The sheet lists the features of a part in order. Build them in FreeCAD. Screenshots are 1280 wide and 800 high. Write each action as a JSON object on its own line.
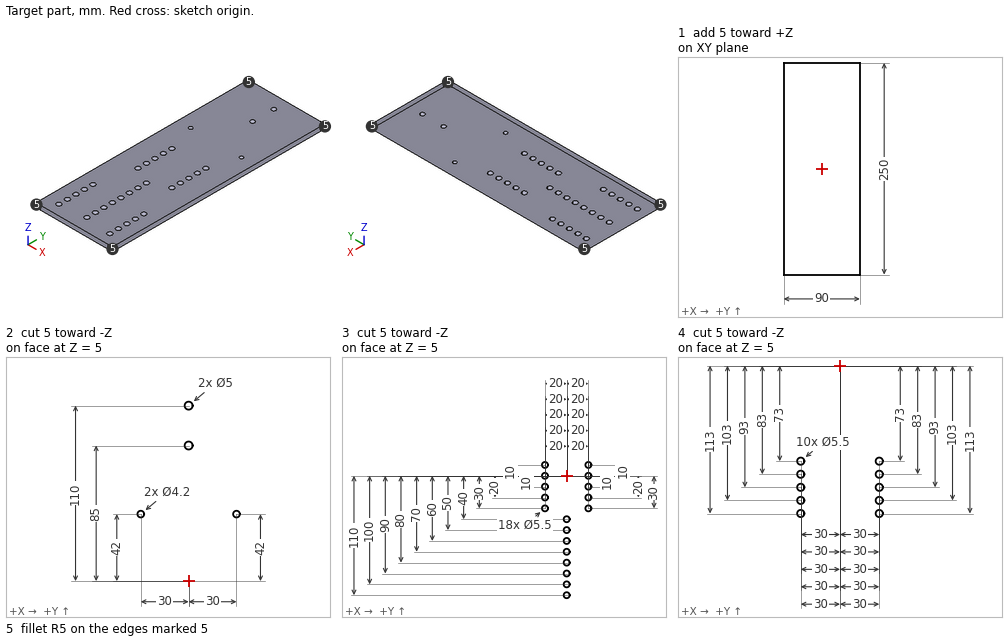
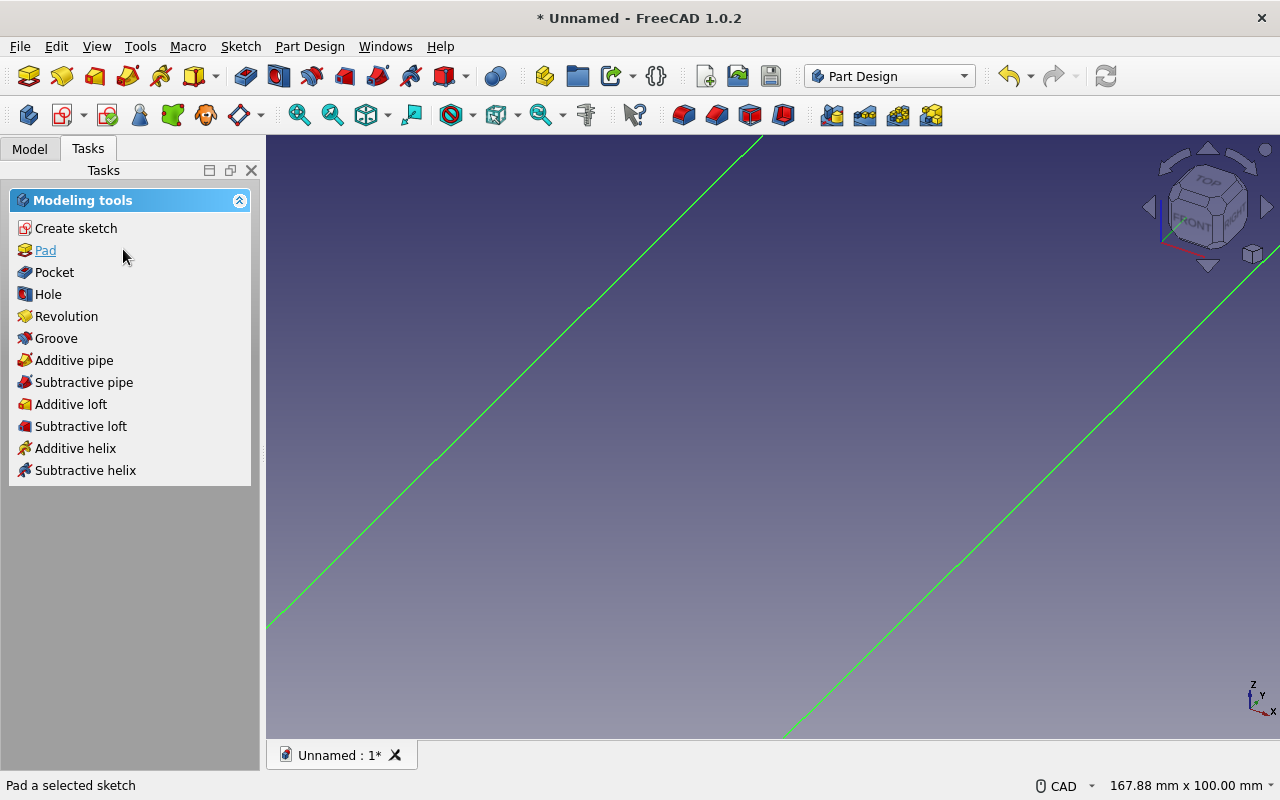
{"action": "left_click", "coordinate": [29, 76]}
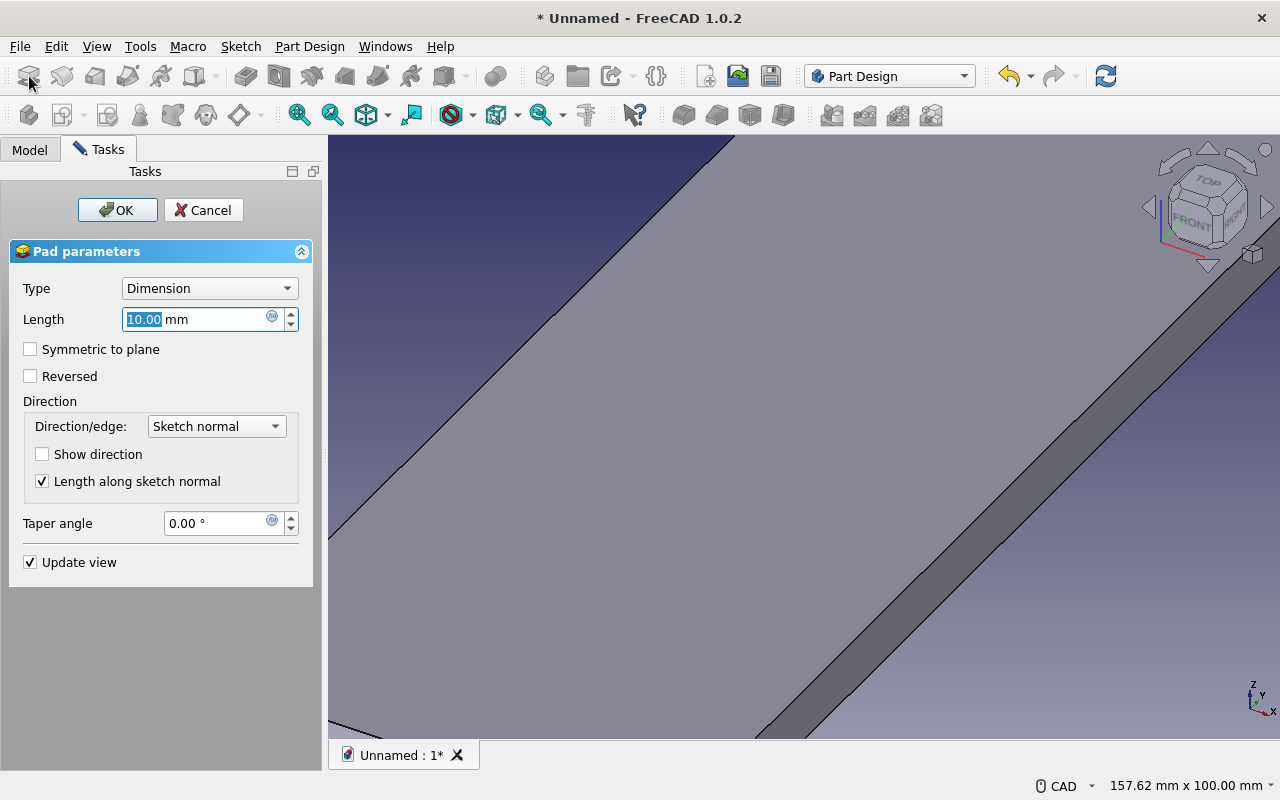
{"action": "type", "text": "5"}
{"action": "key", "text": "Tab"}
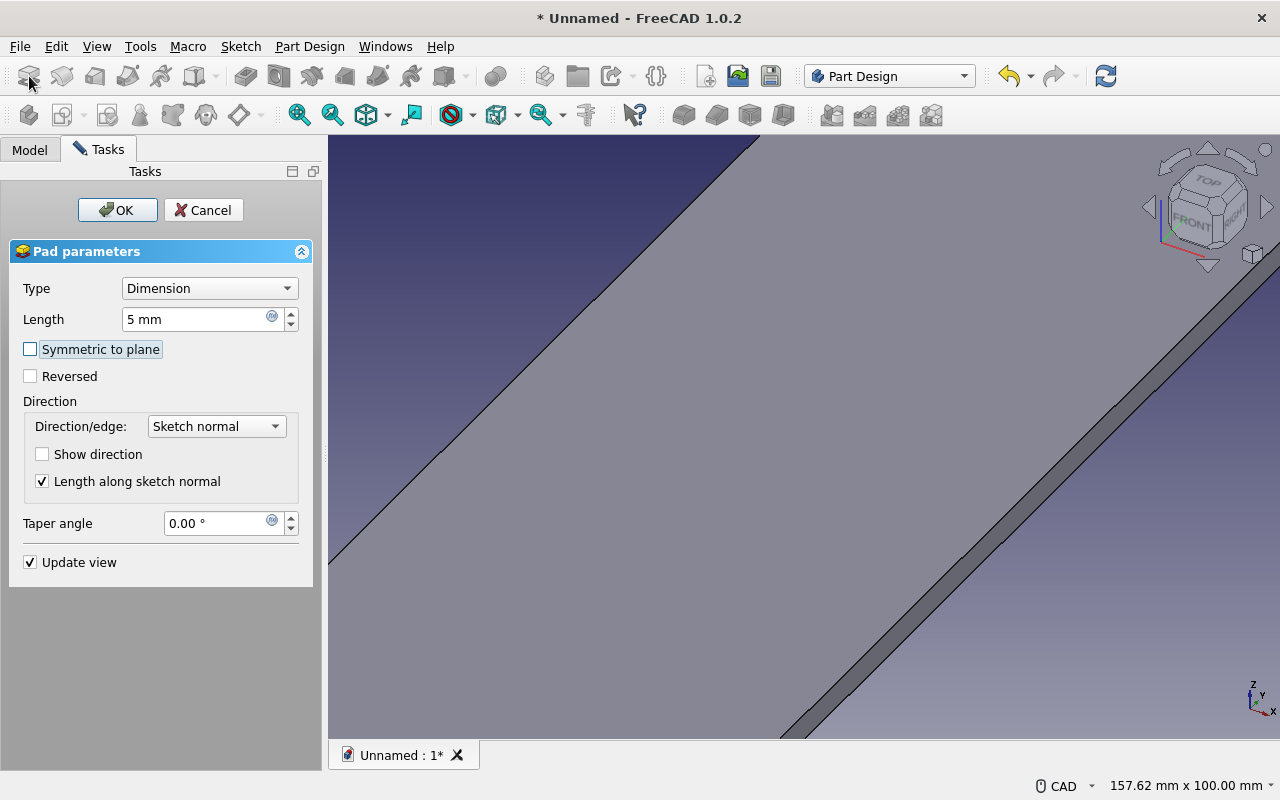
{"action": "left_click", "coordinate": [118, 210]}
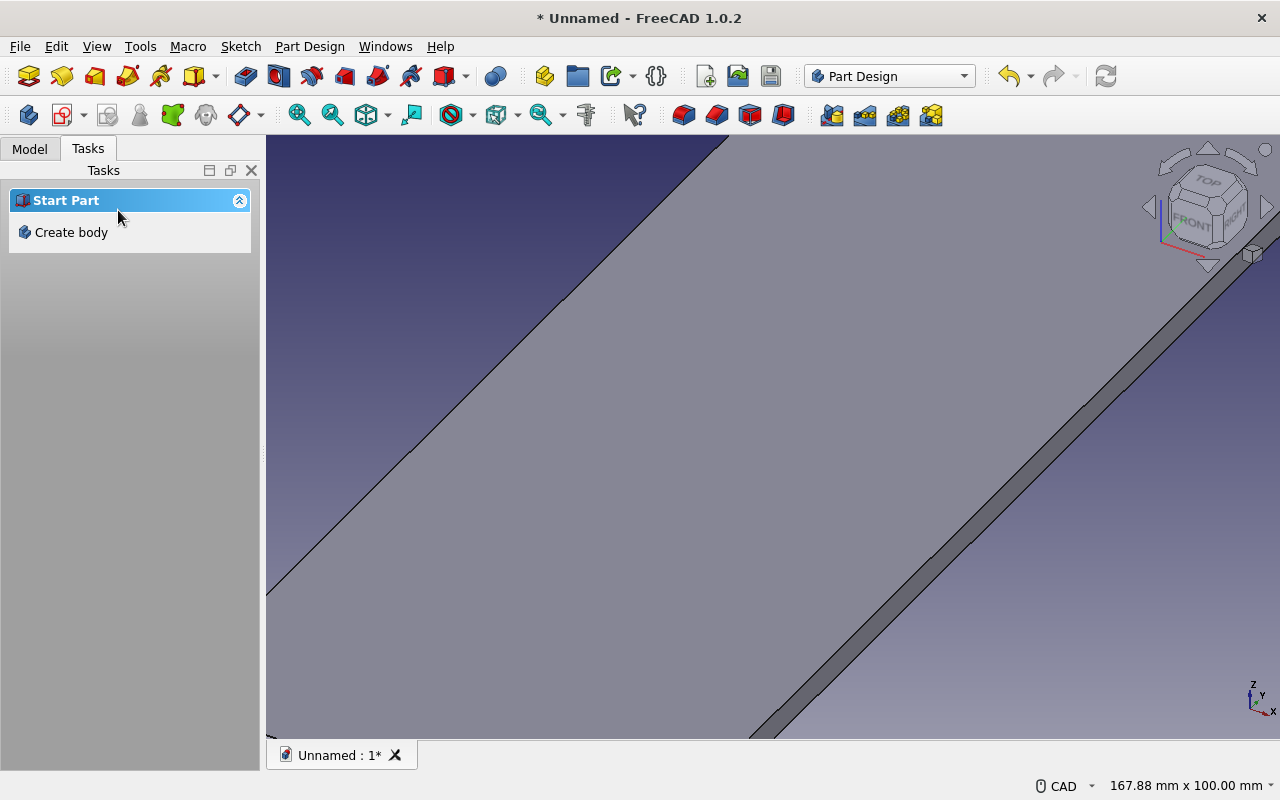
{"action": "key", "text": "v f"}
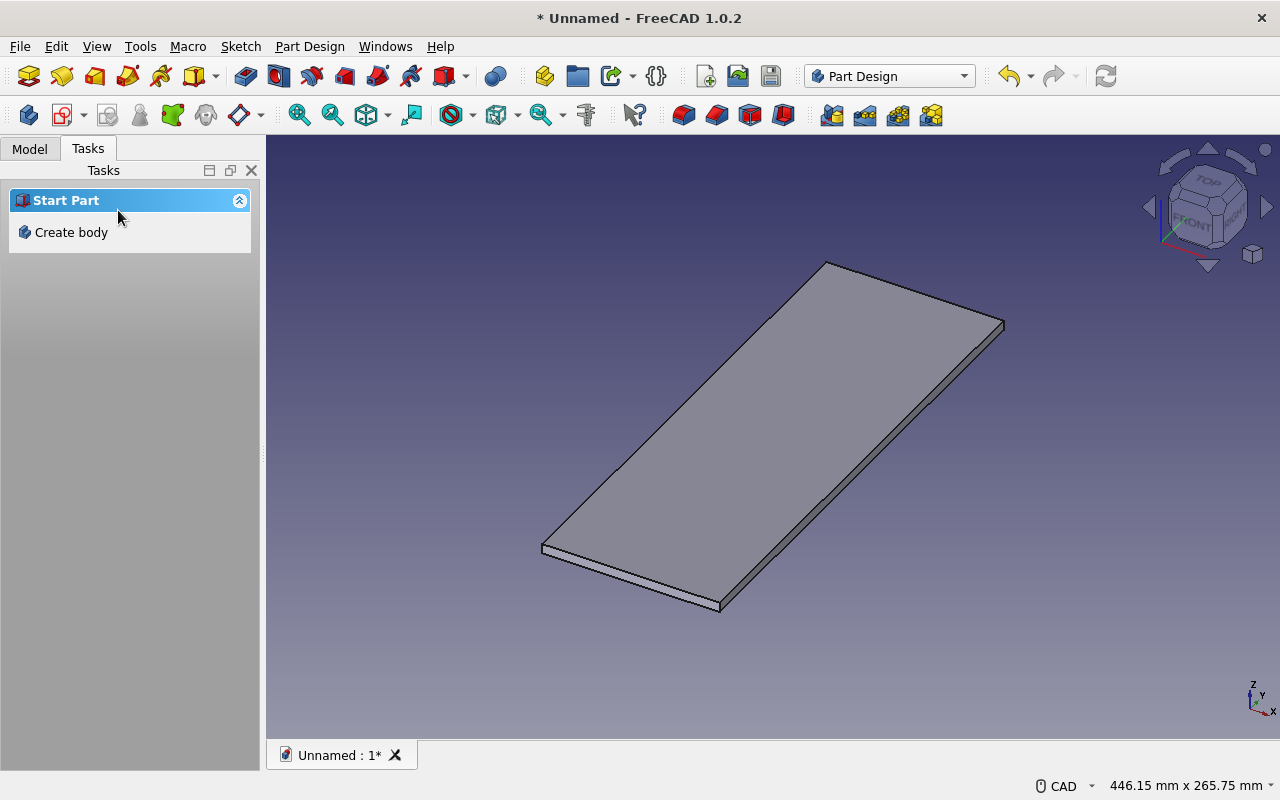
{"action": "left_click", "coordinate": [854, 351]}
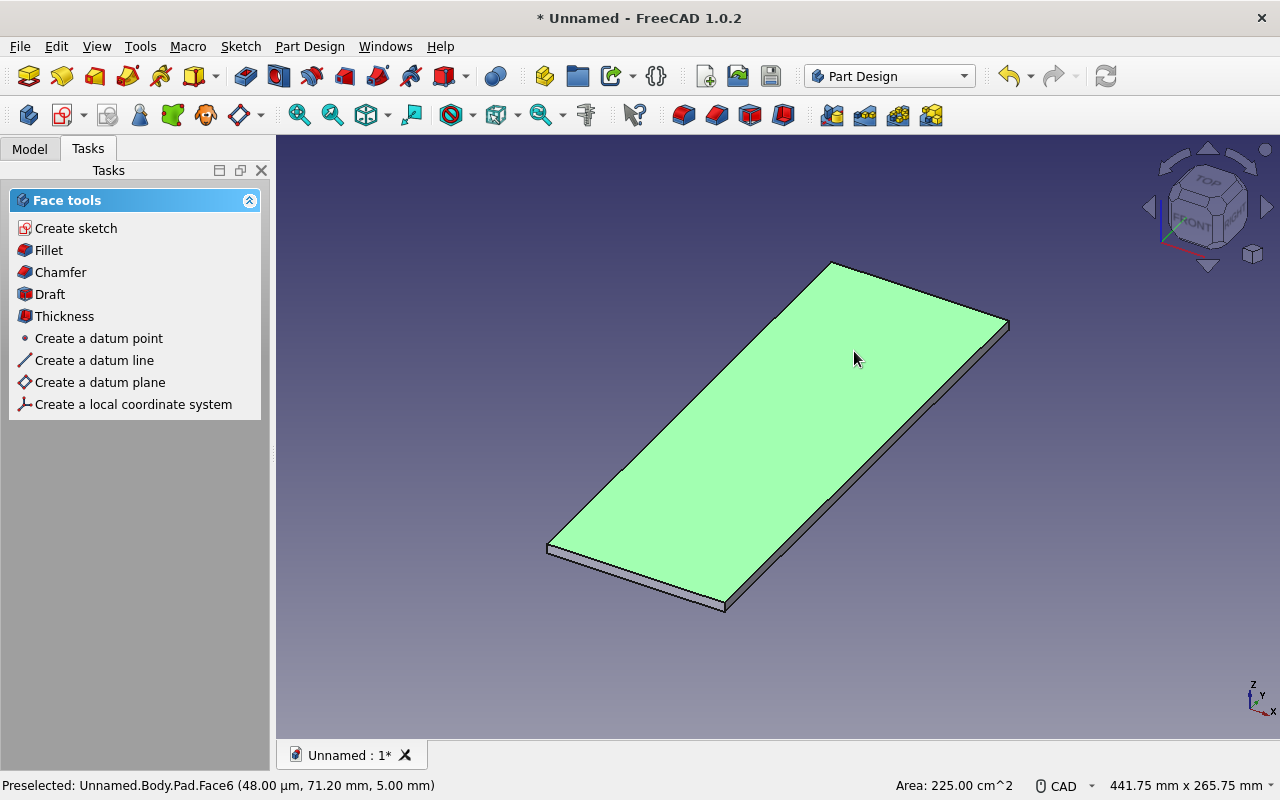
{"action": "left_click", "coordinate": [62, 116]}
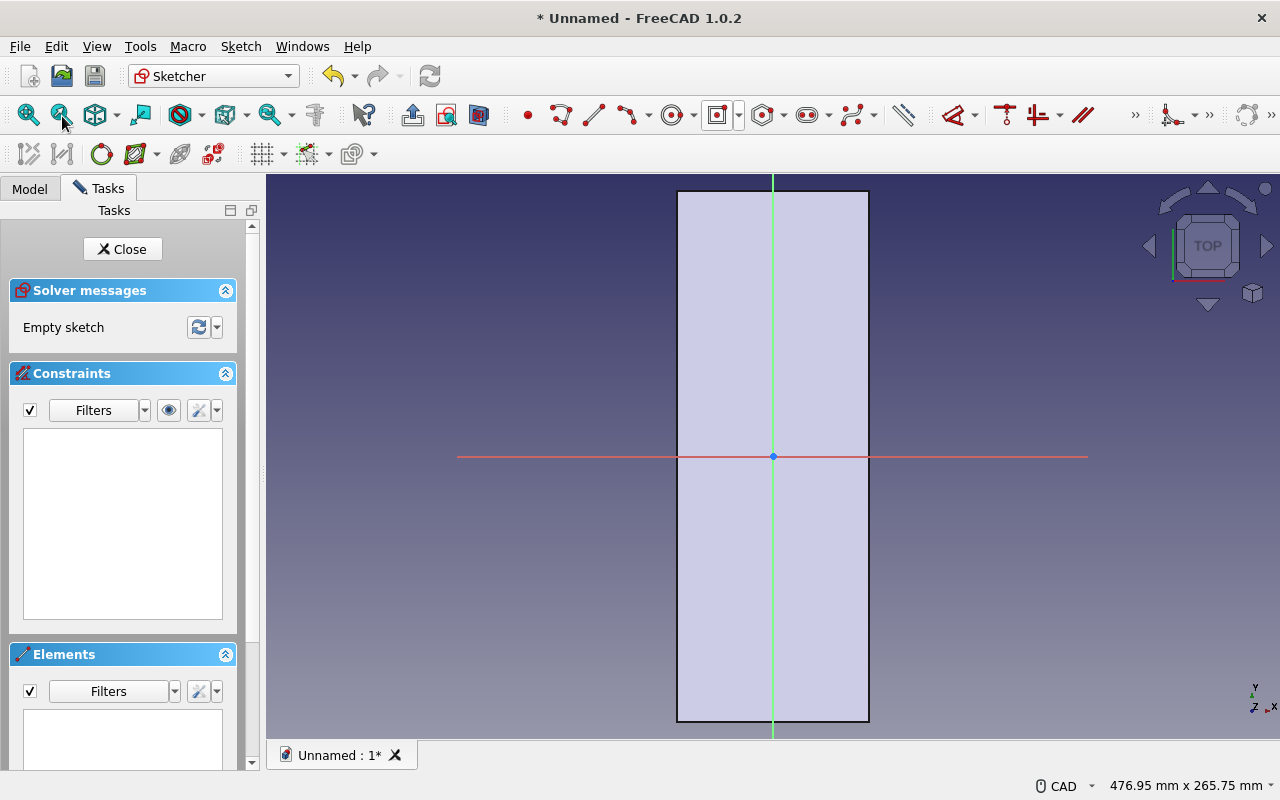
{"action": "scroll", "coordinate": [395, 711], "scroll_direction": "down", "scroll_amount": 1}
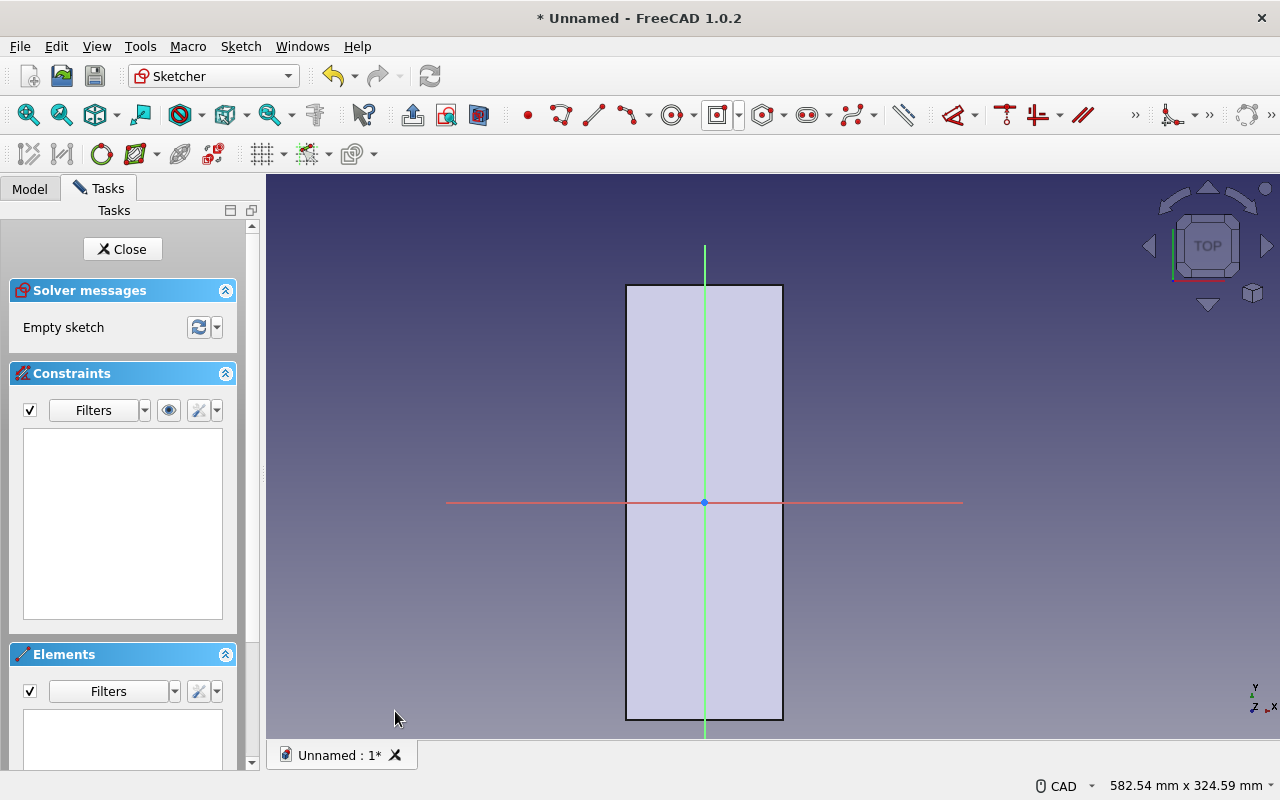
{"action": "scroll", "coordinate": [705, 342], "scroll_direction": "up", "scroll_amount": 3}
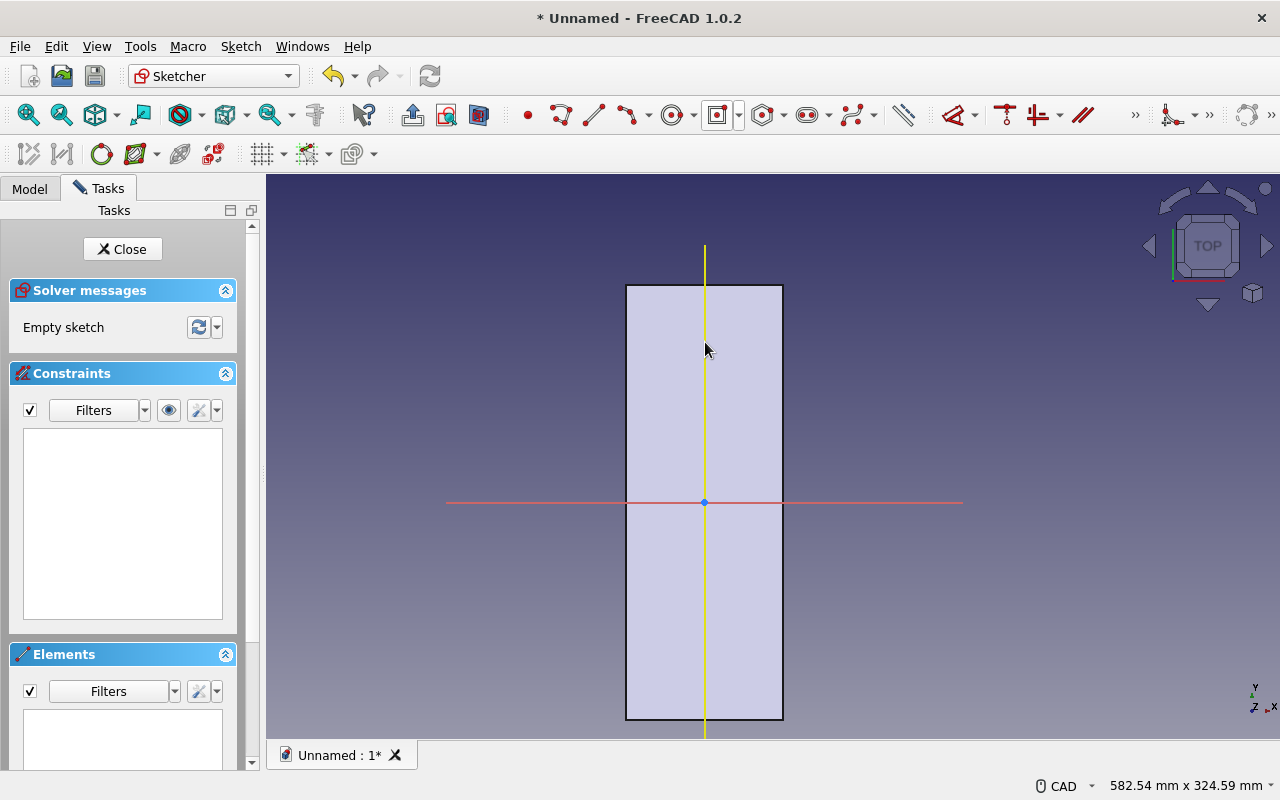
{"action": "key", "text": "g c"}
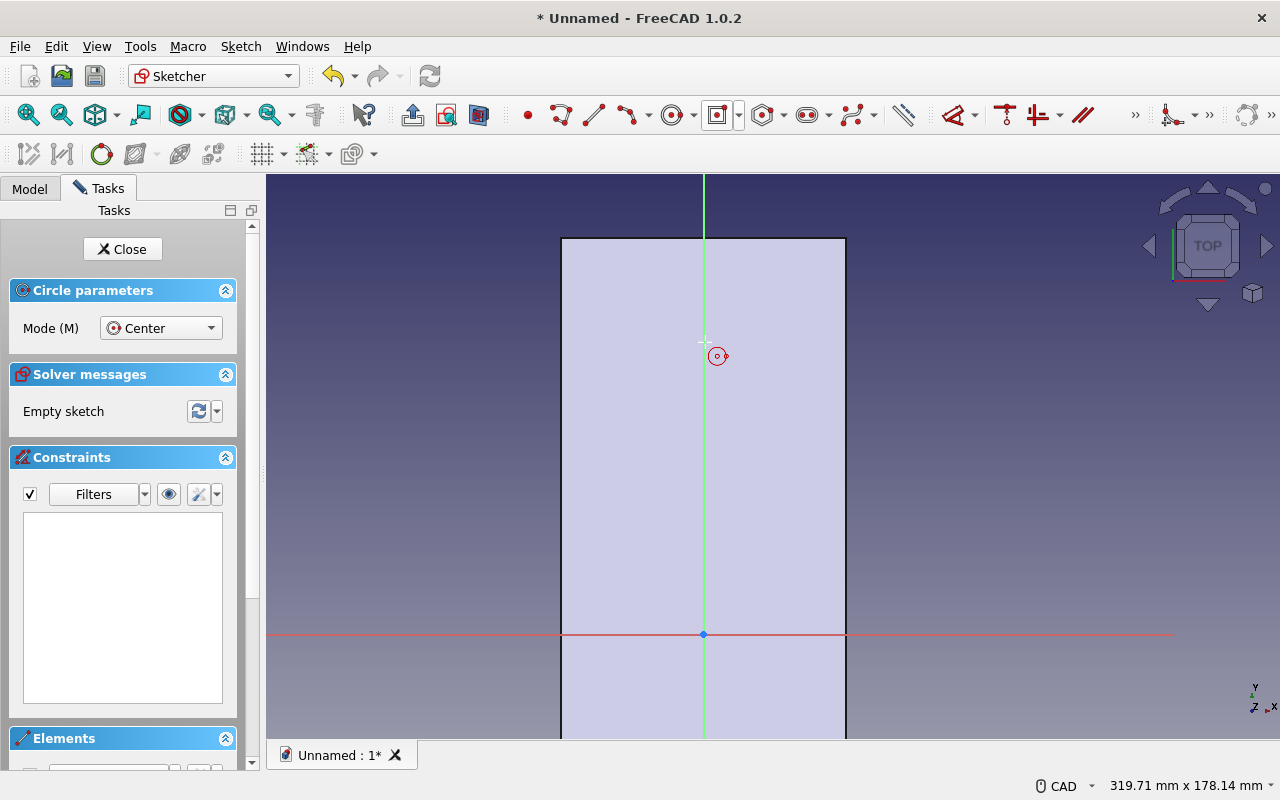
{"action": "scroll", "coordinate": [704, 286], "scroll_direction": "up", "scroll_amount": 6}